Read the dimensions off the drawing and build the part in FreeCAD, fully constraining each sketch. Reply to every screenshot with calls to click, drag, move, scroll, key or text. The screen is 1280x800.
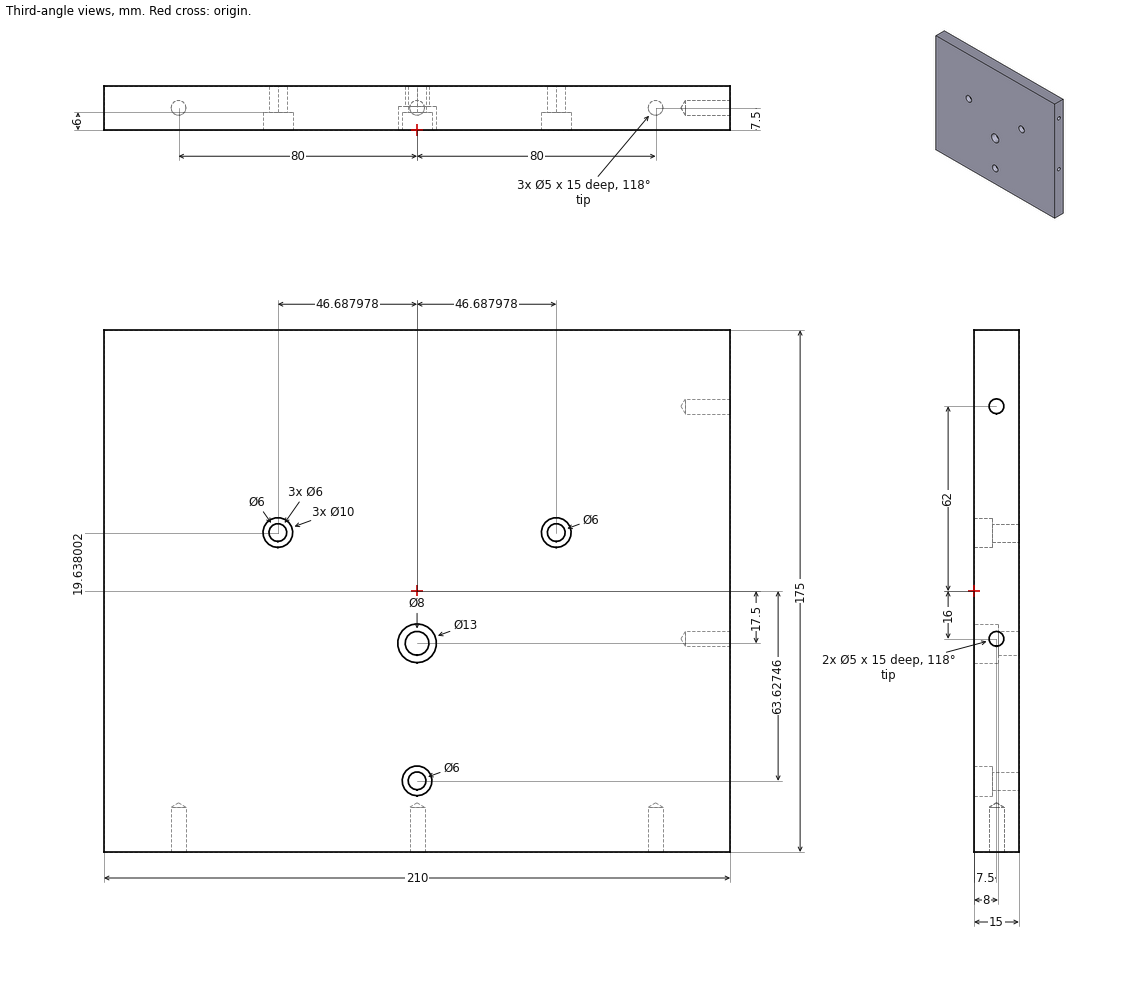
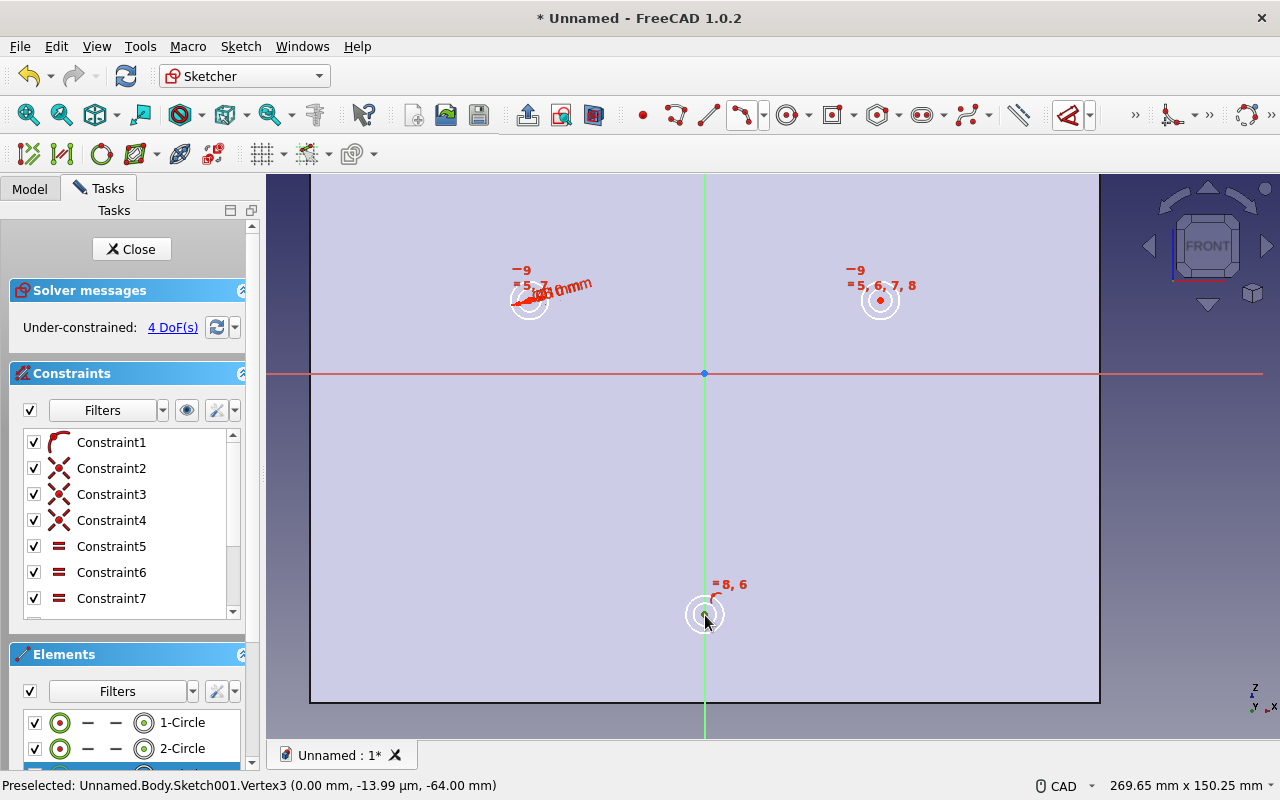
click(1090, 116)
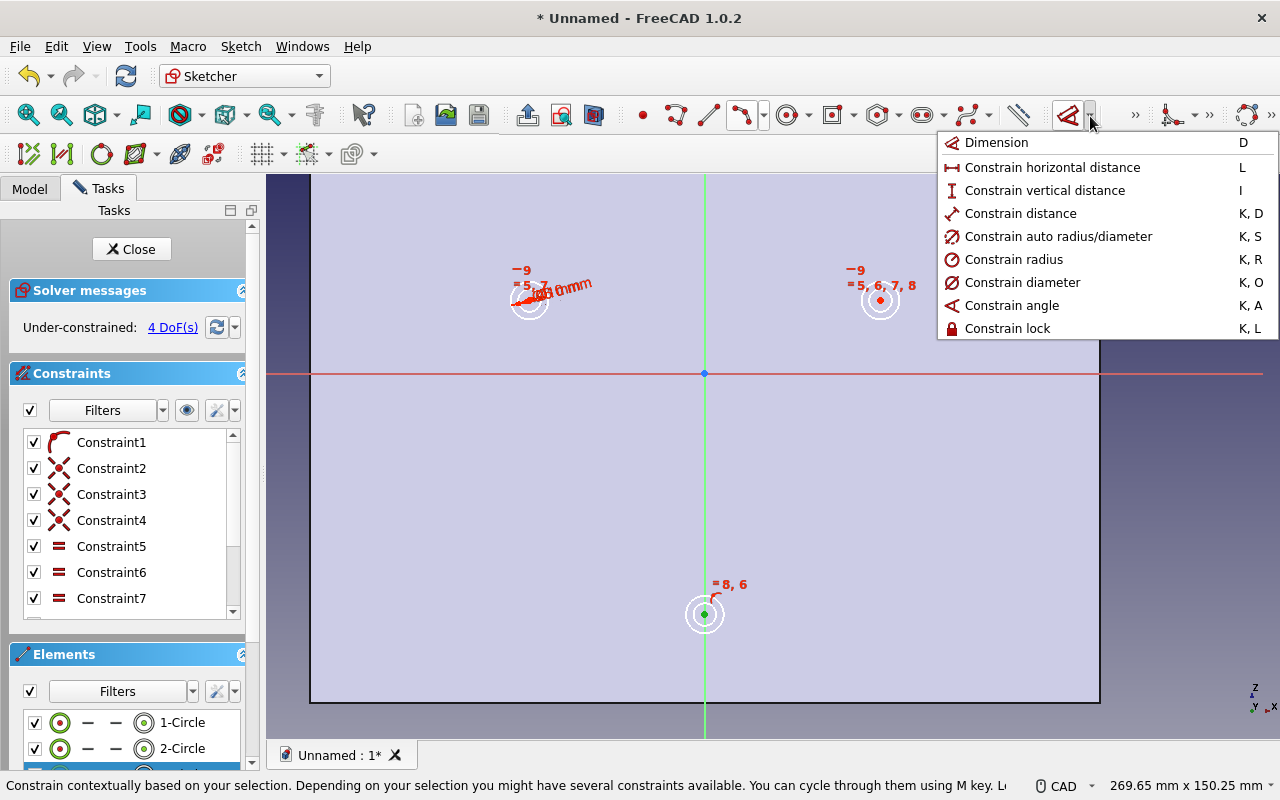
click(1108, 190)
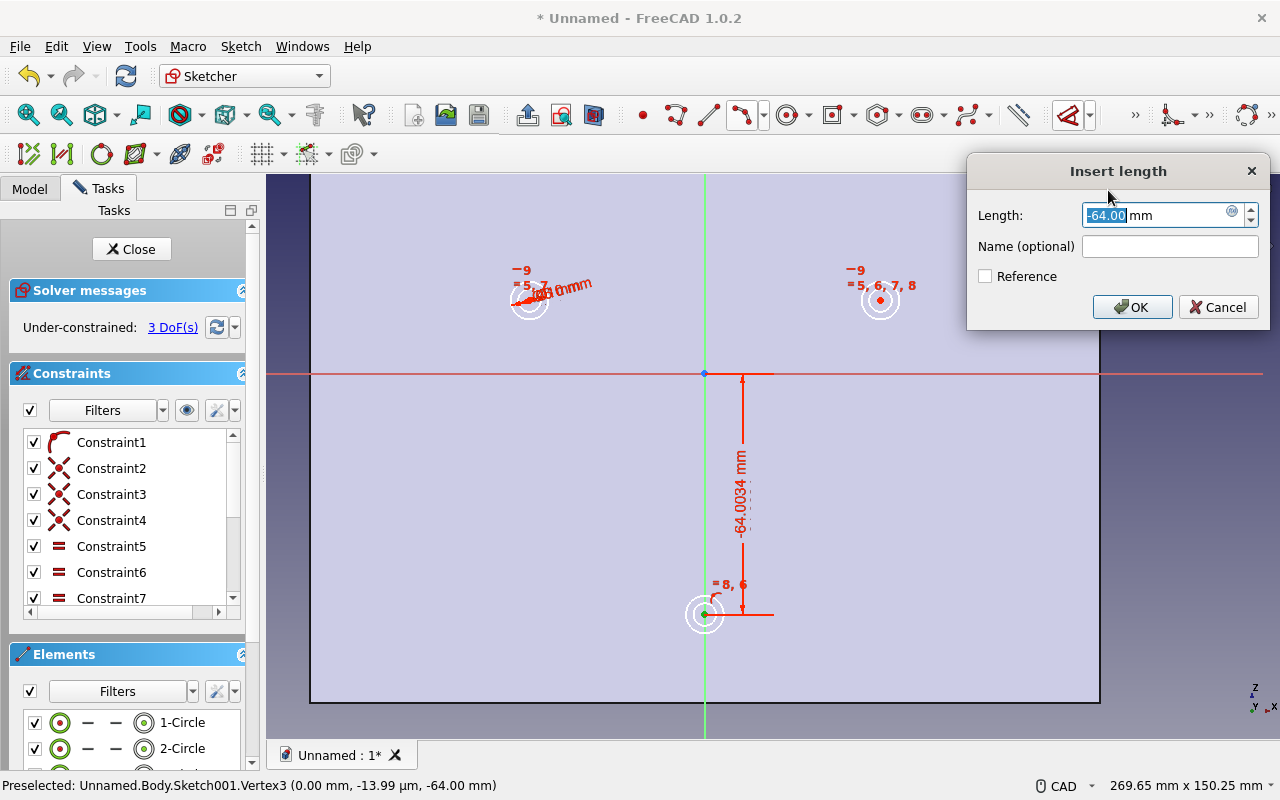
text(-63.62746)
key(Return)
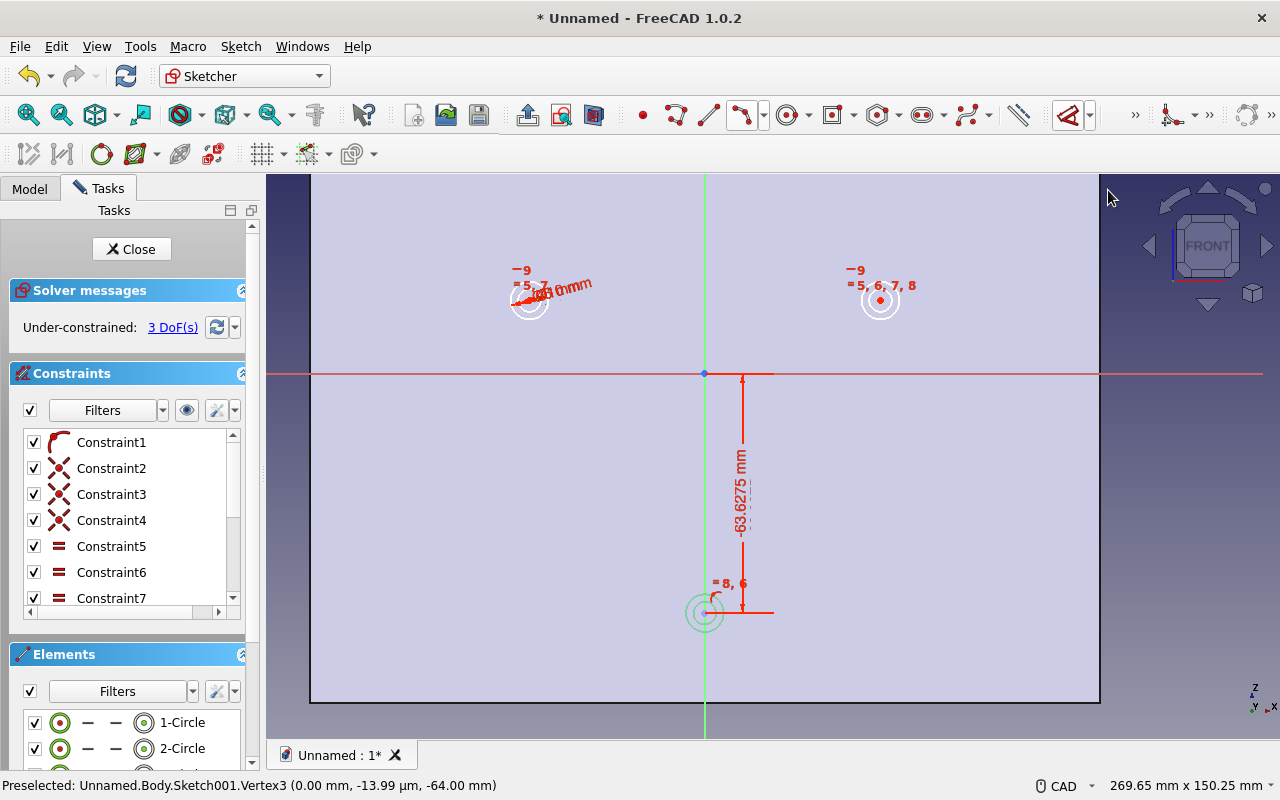
click(530, 301)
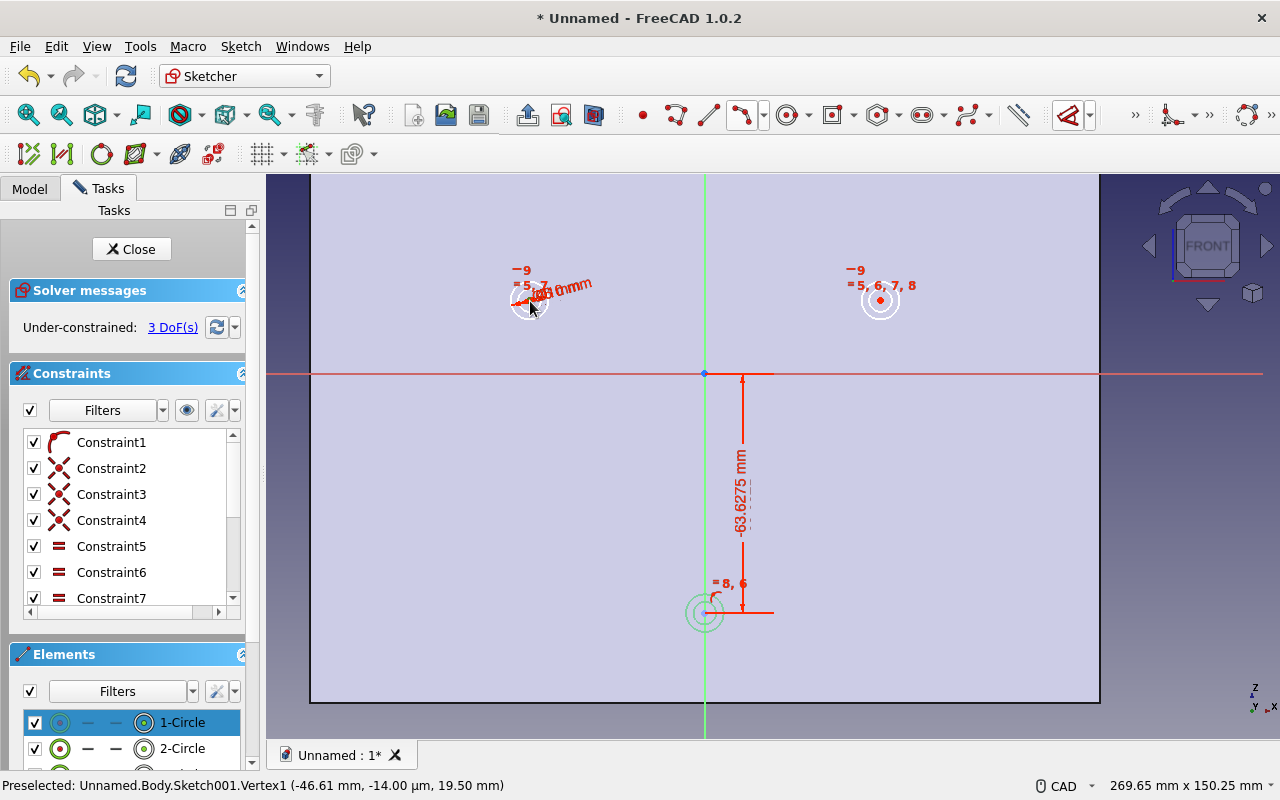
click(1090, 116)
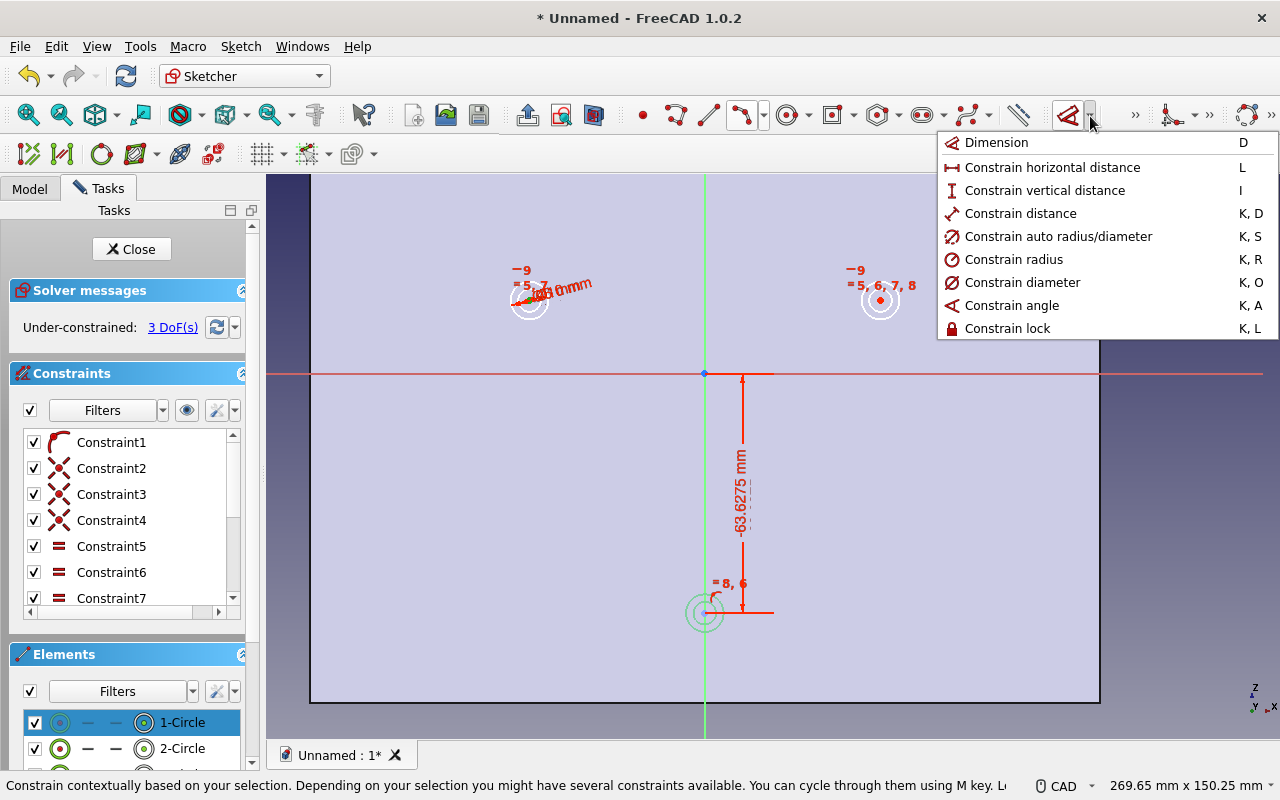
click(1108, 168)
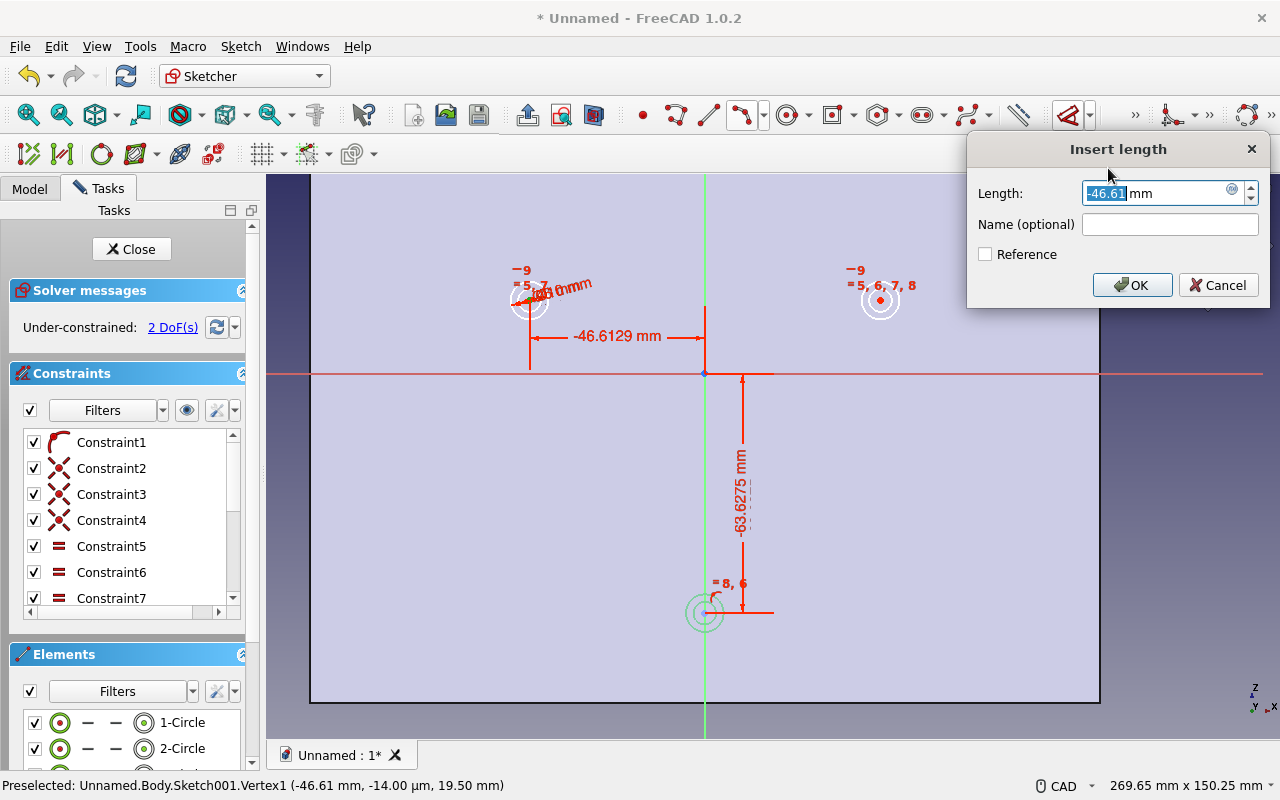
text(-46.687978)
key(Return)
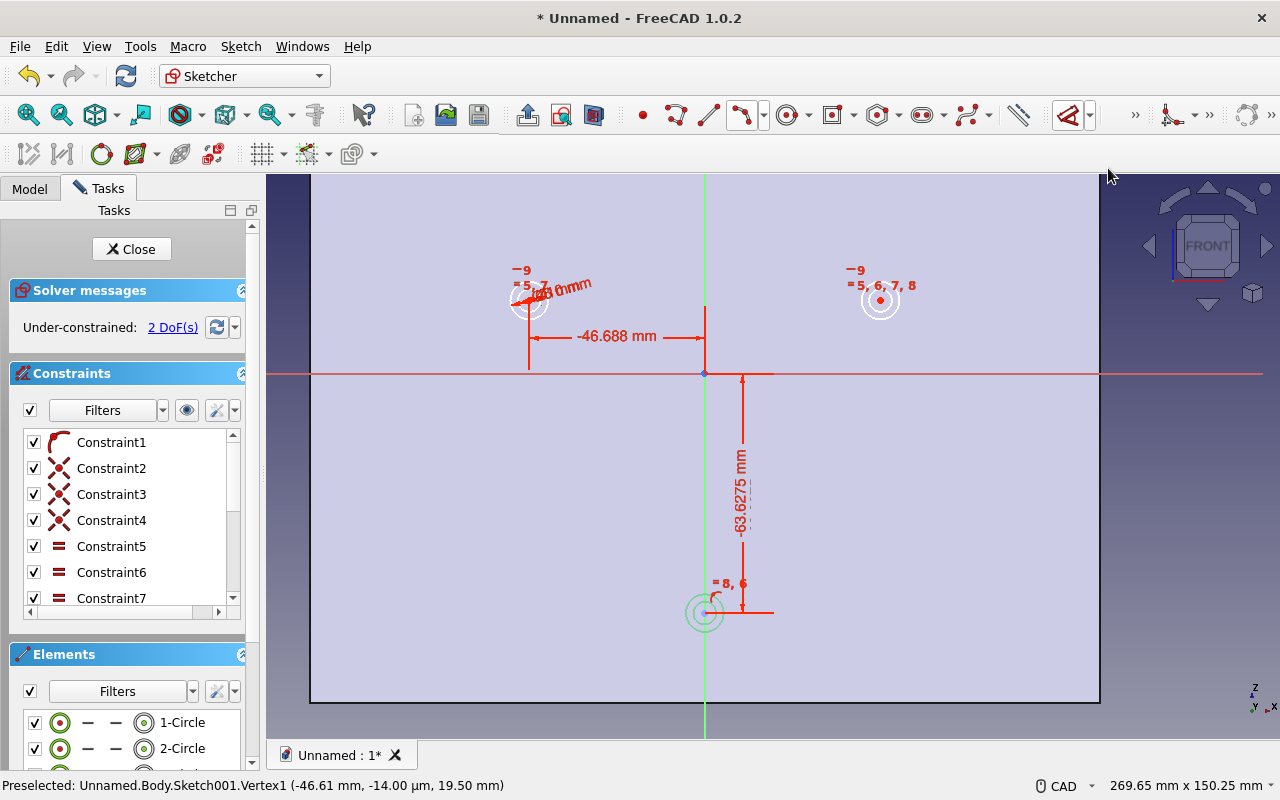
click(529, 301)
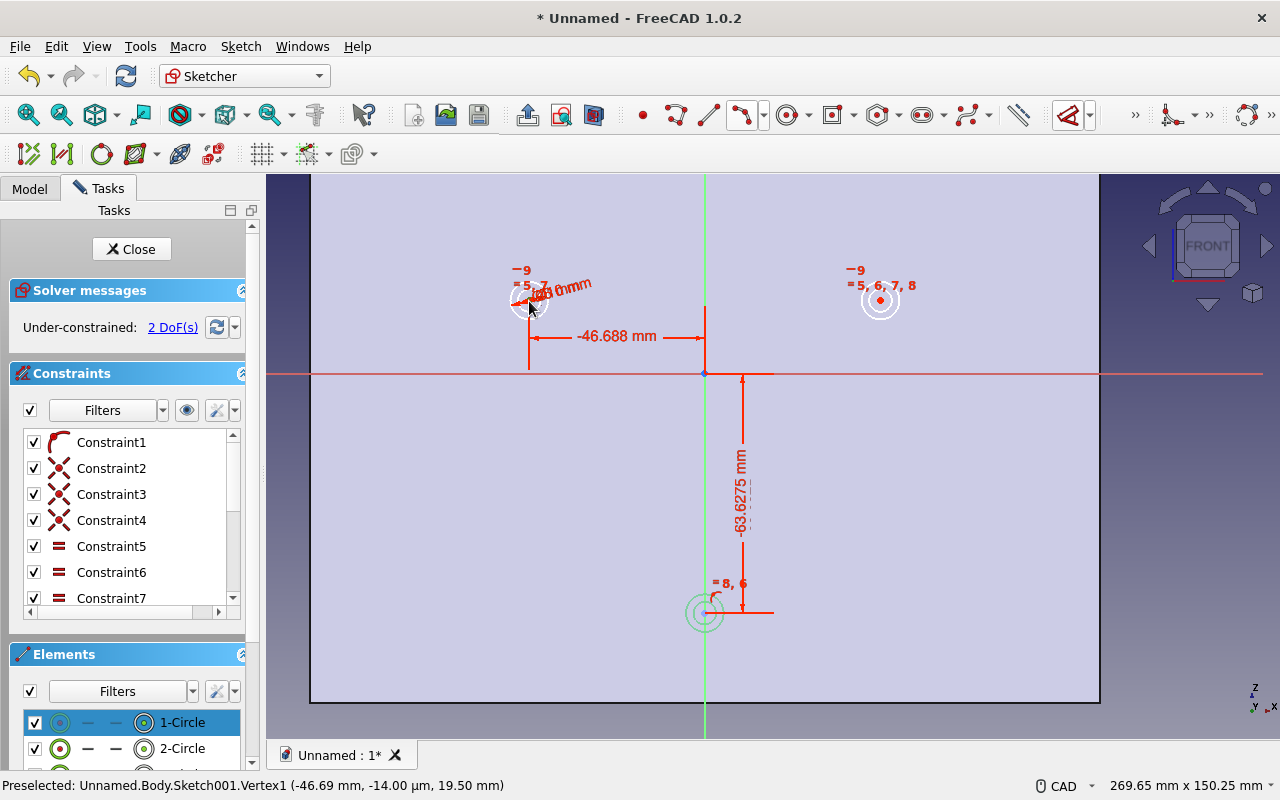
key(i)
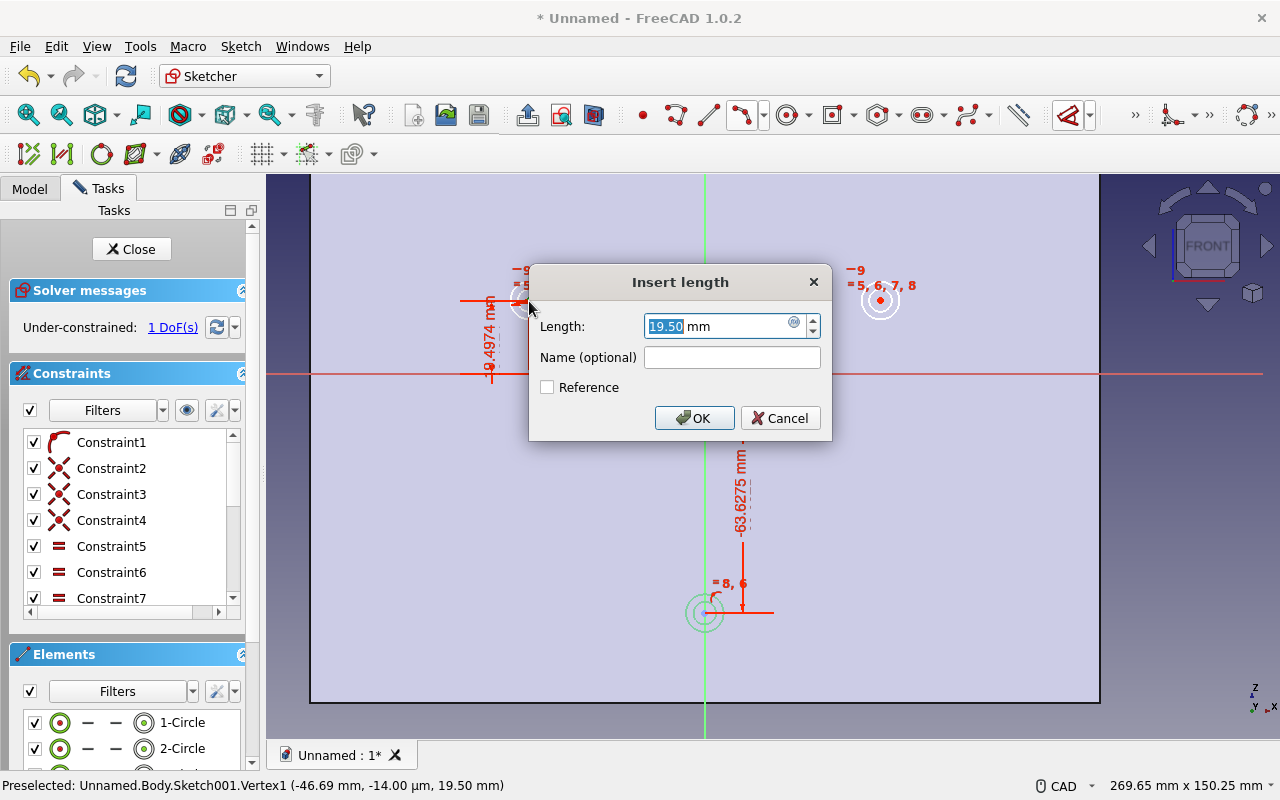
text(19.638002)
key(Return)